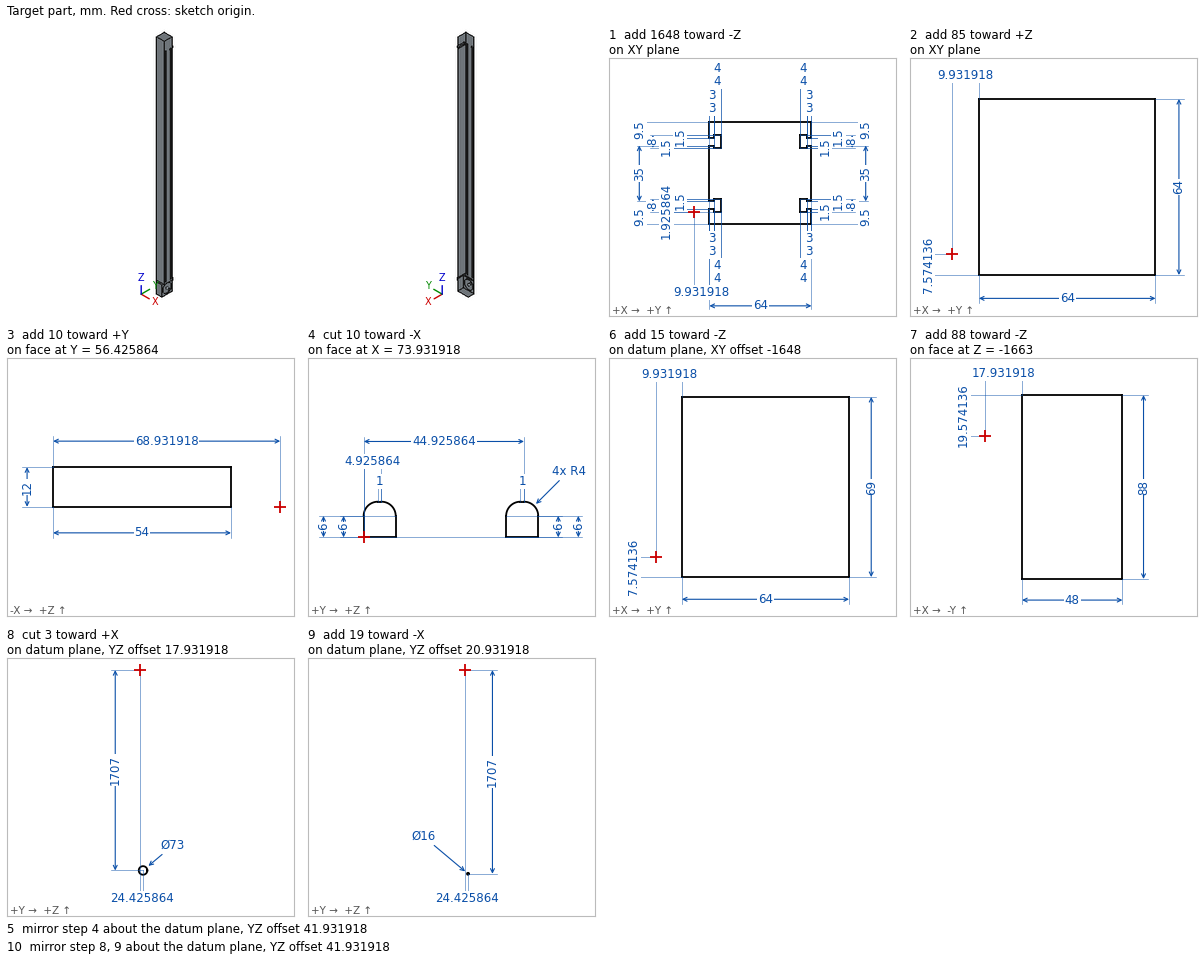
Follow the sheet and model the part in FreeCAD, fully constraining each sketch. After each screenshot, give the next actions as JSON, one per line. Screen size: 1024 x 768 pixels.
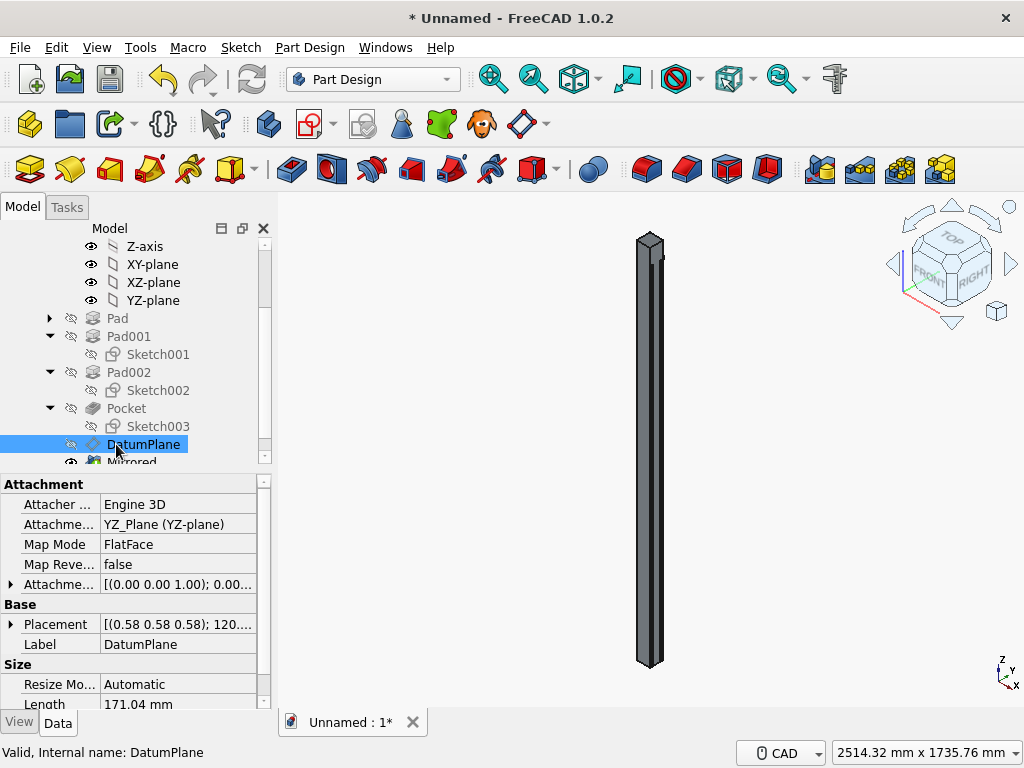
{"action": "key", "text": "5"}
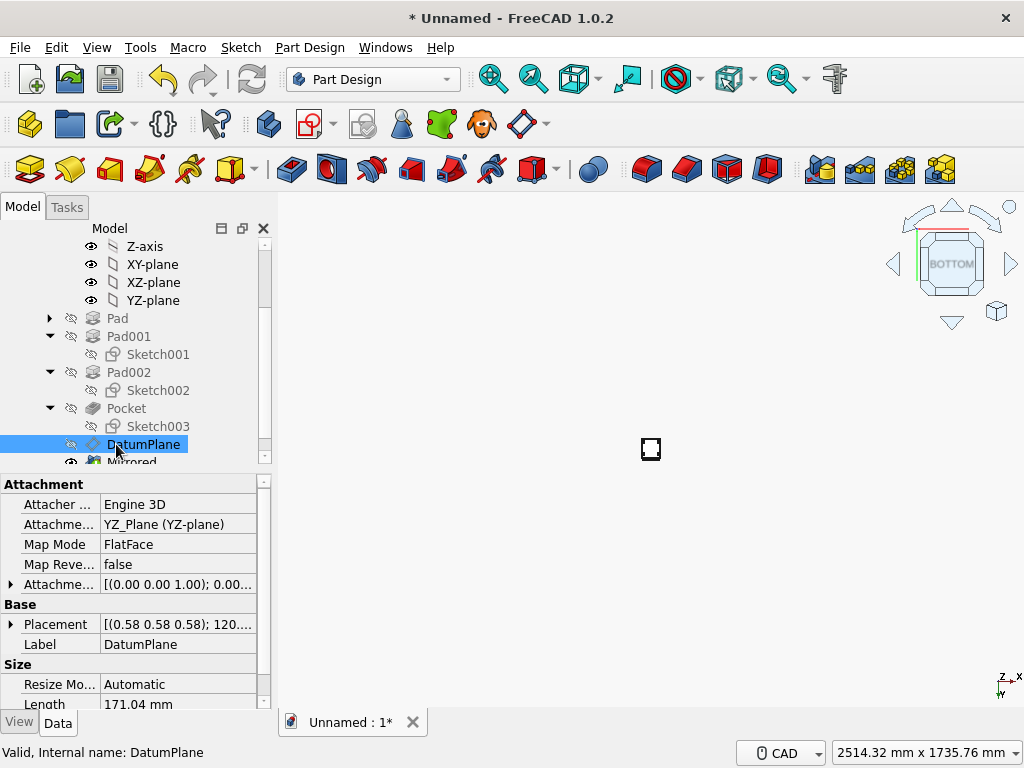
{"action": "left_click", "coordinate": [494, 80]}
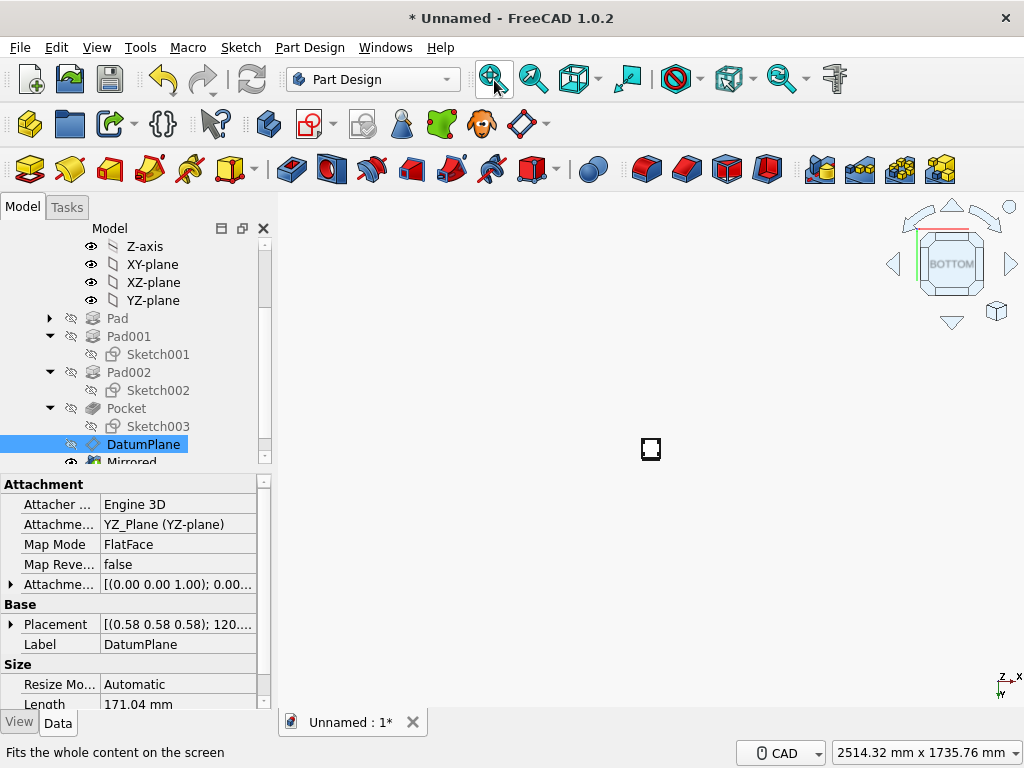
{"action": "key", "text": "1"}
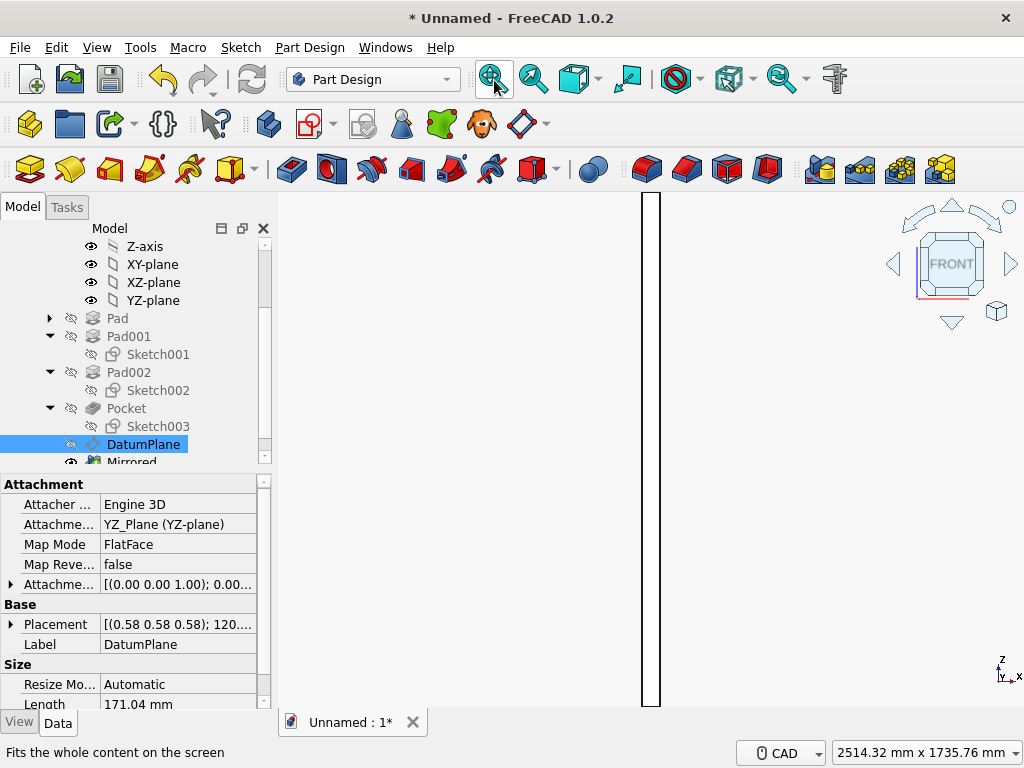
{"action": "left_click", "coordinate": [494, 80]}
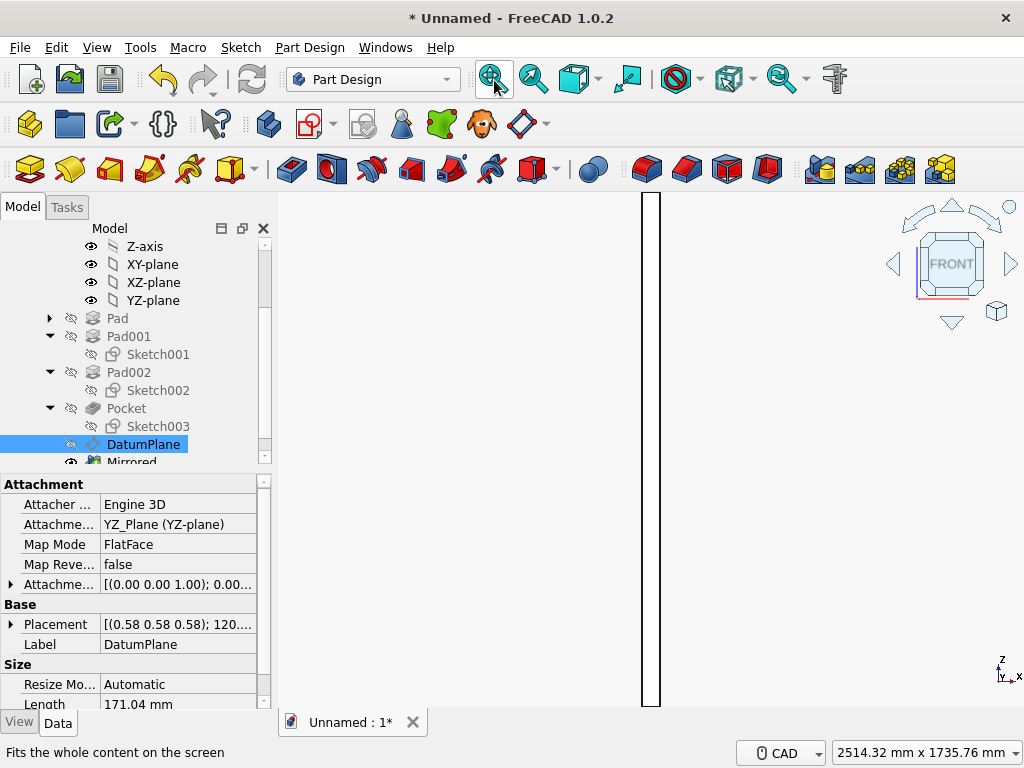
{"action": "key", "text": "3"}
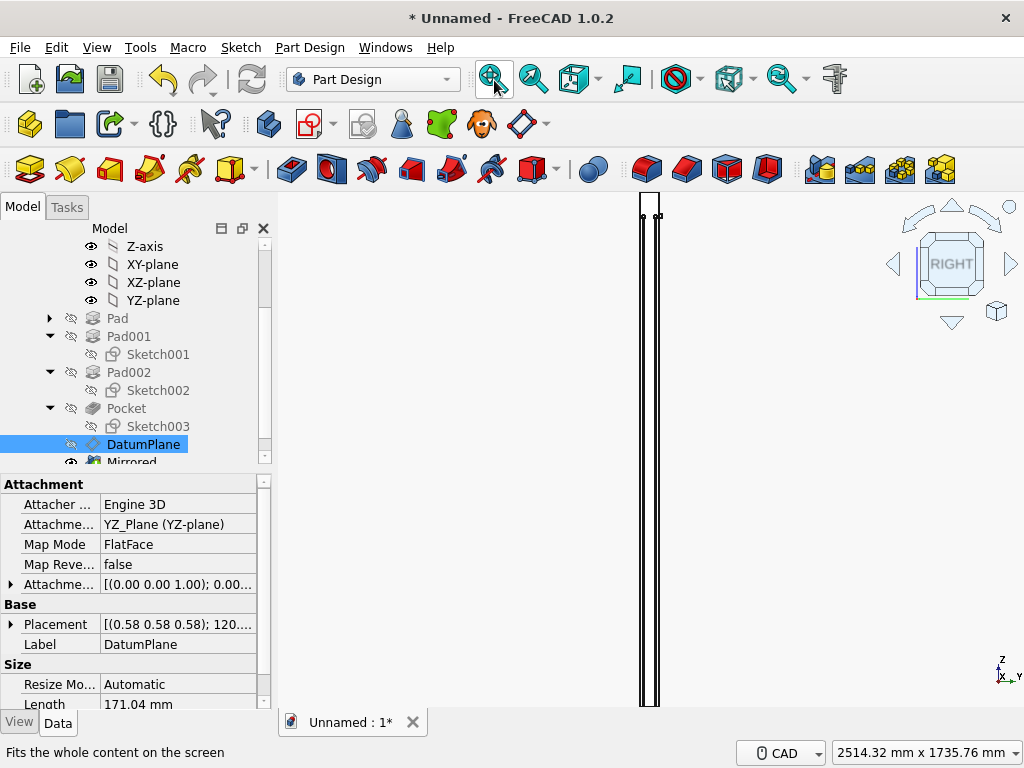
{"action": "left_click", "coordinate": [494, 80]}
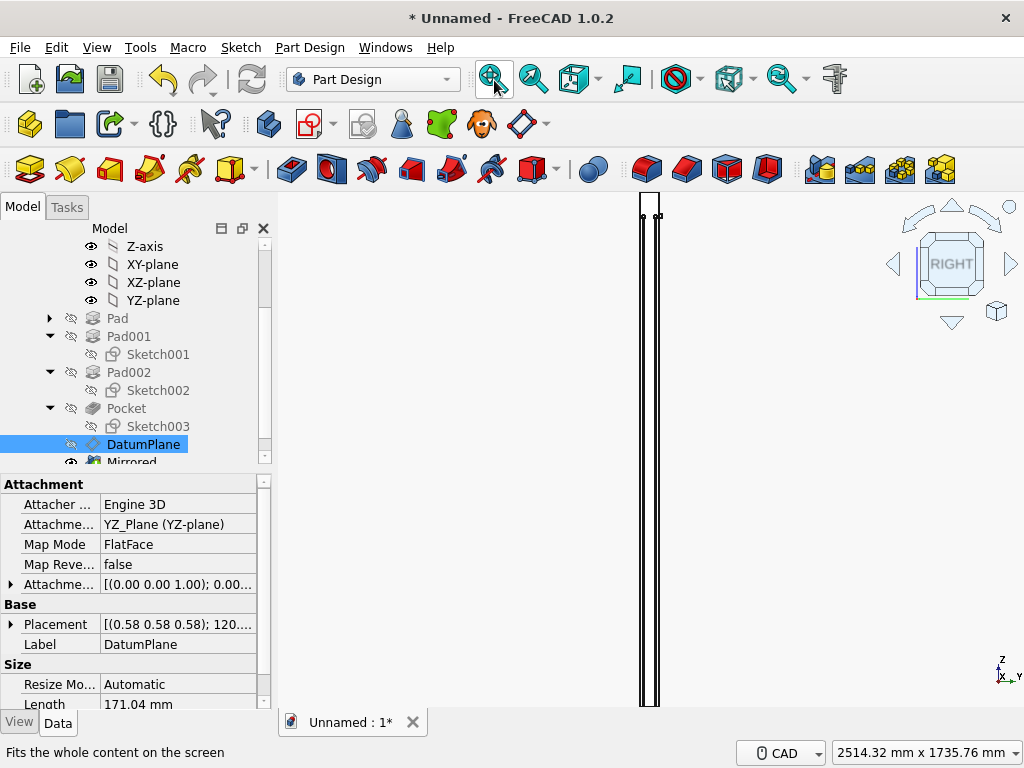
{"action": "scroll", "coordinate": [160, 350], "scroll_direction": "down", "scroll_amount": 3}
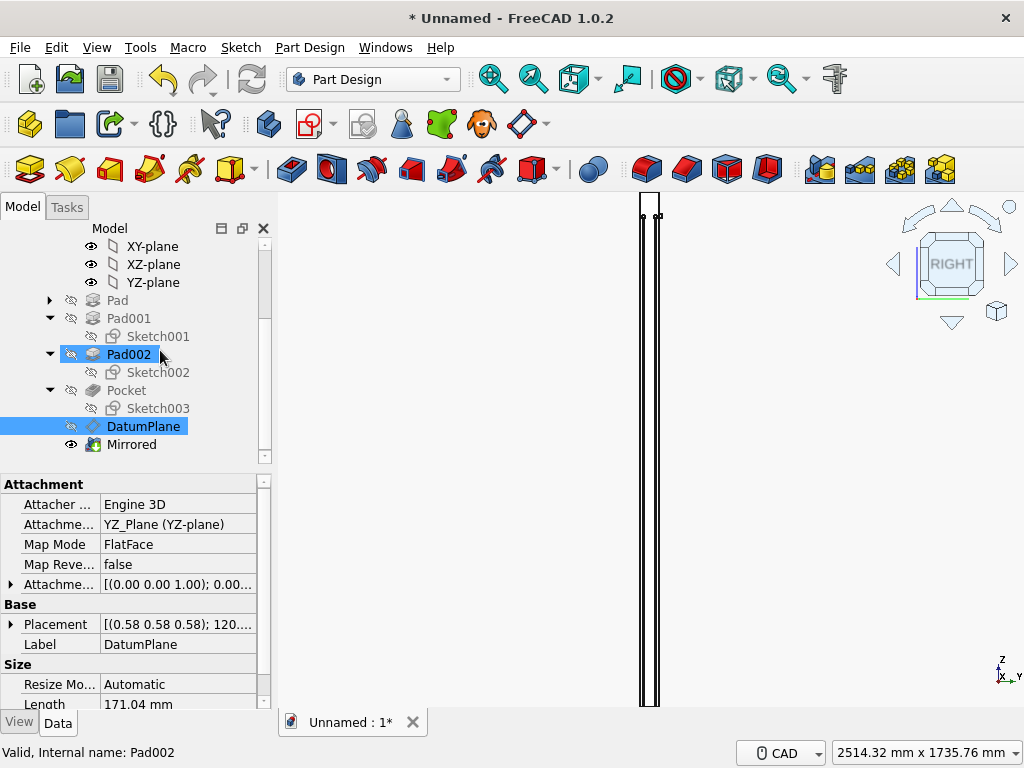
{"action": "scroll", "coordinate": [160, 350], "scroll_direction": "up", "scroll_amount": 15}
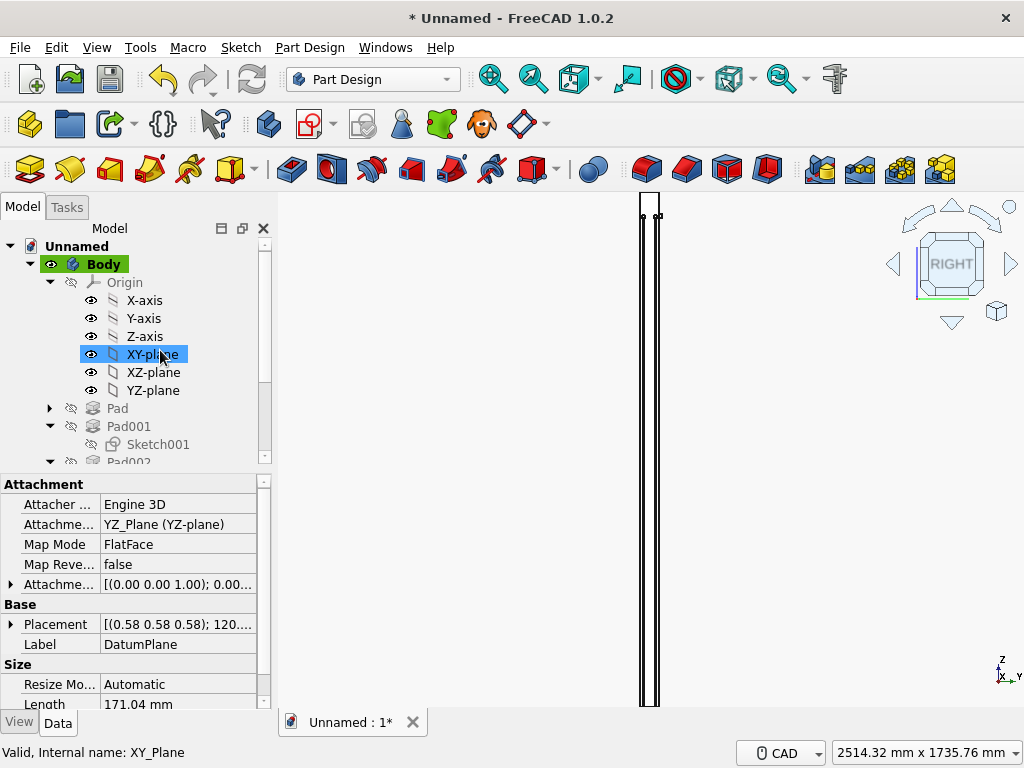
{"action": "left_click", "coordinate": [136, 354]}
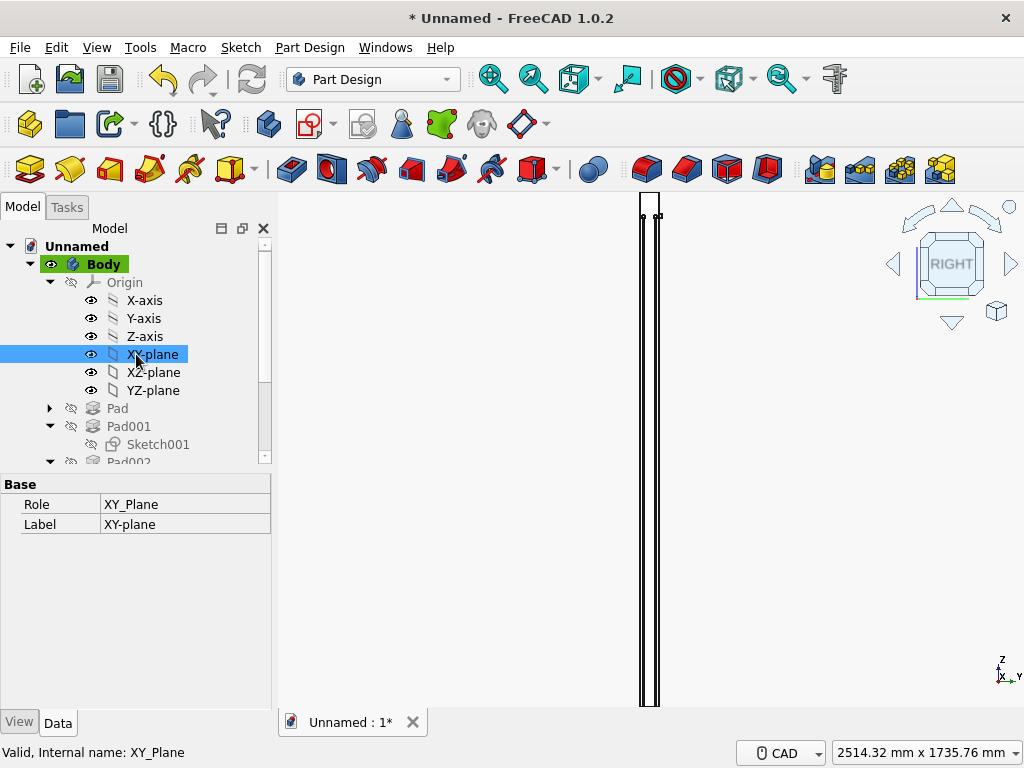
{"action": "left_click", "coordinate": [522, 124]}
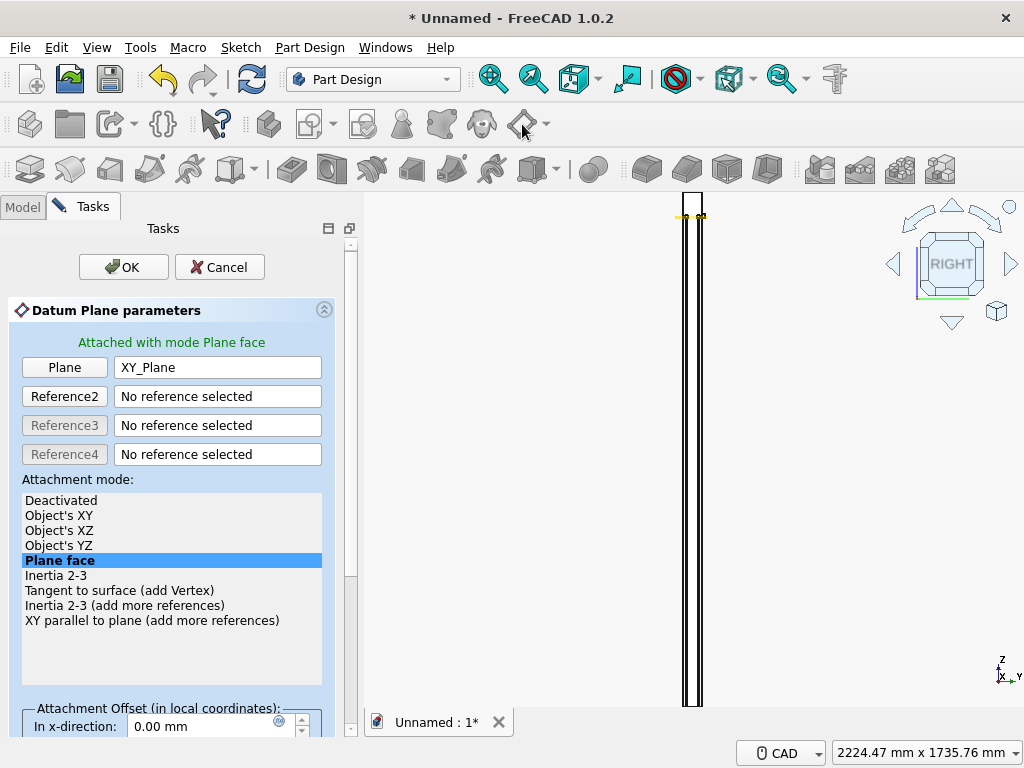
{"action": "scroll", "coordinate": [351, 487], "scroll_direction": "down", "scroll_amount": 3}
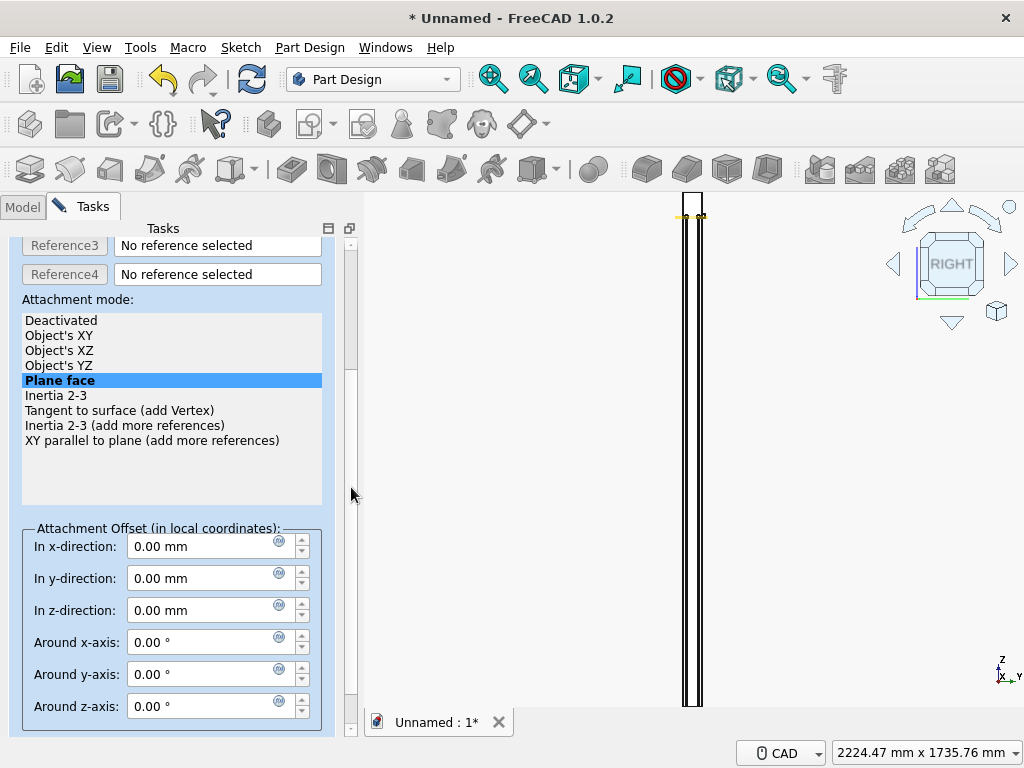
{"action": "triple_click", "coordinate": [210, 610]}